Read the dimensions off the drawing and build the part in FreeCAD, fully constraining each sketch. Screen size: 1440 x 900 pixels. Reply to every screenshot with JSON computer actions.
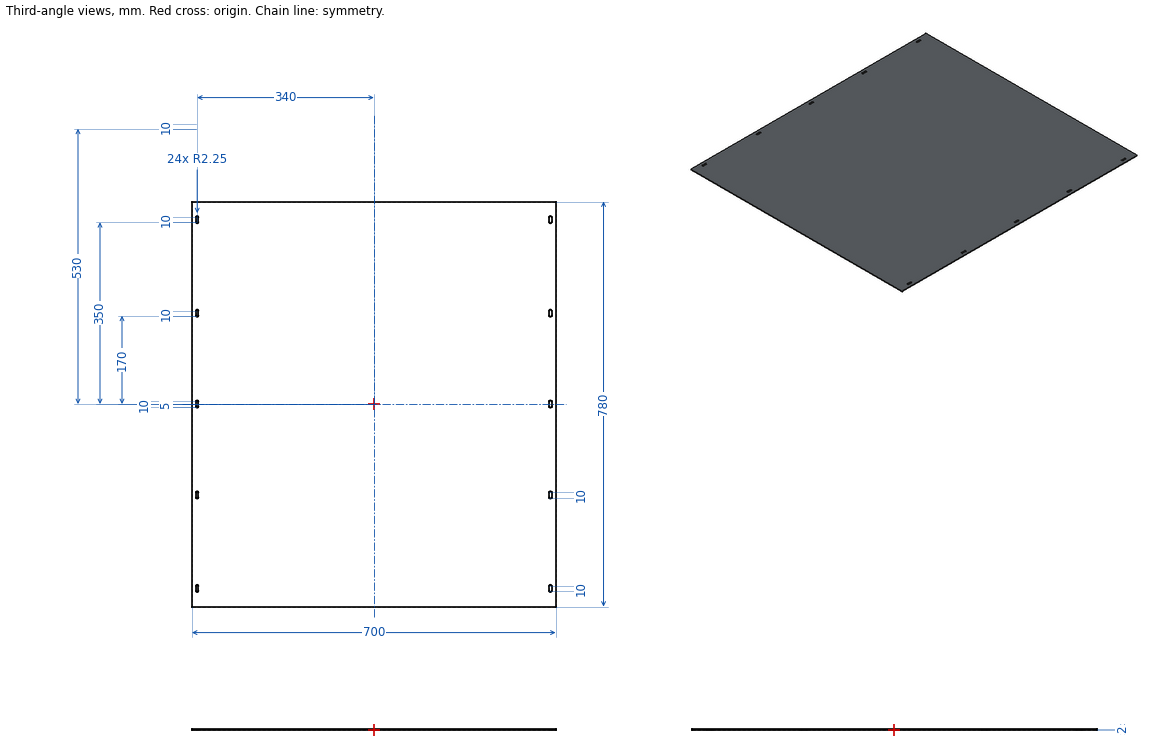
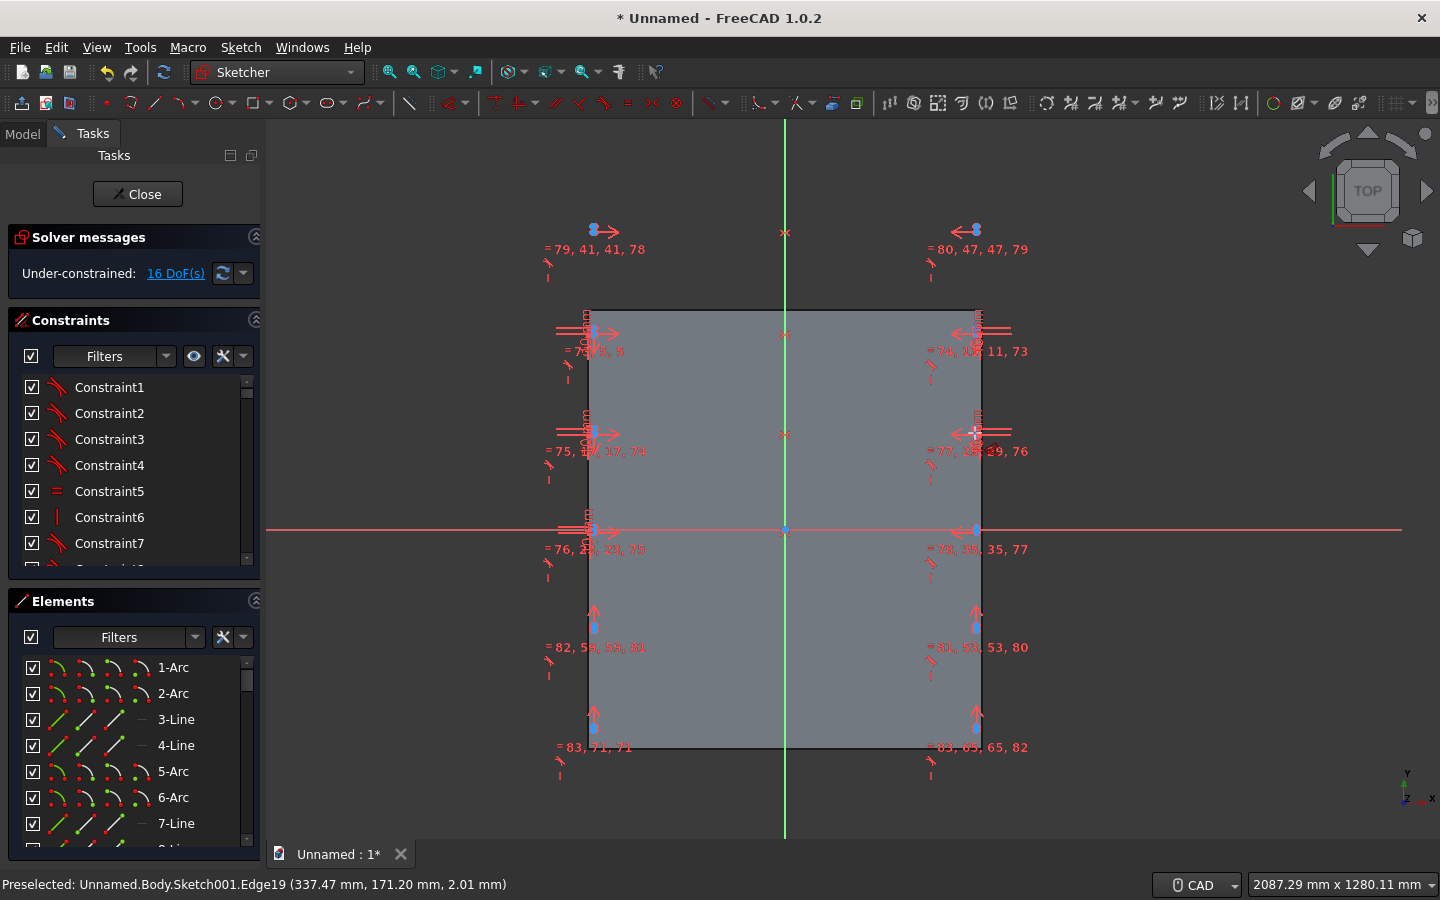
{"action": "scroll", "coordinate": [975, 531], "scroll_direction": "up", "scroll_amount": 12}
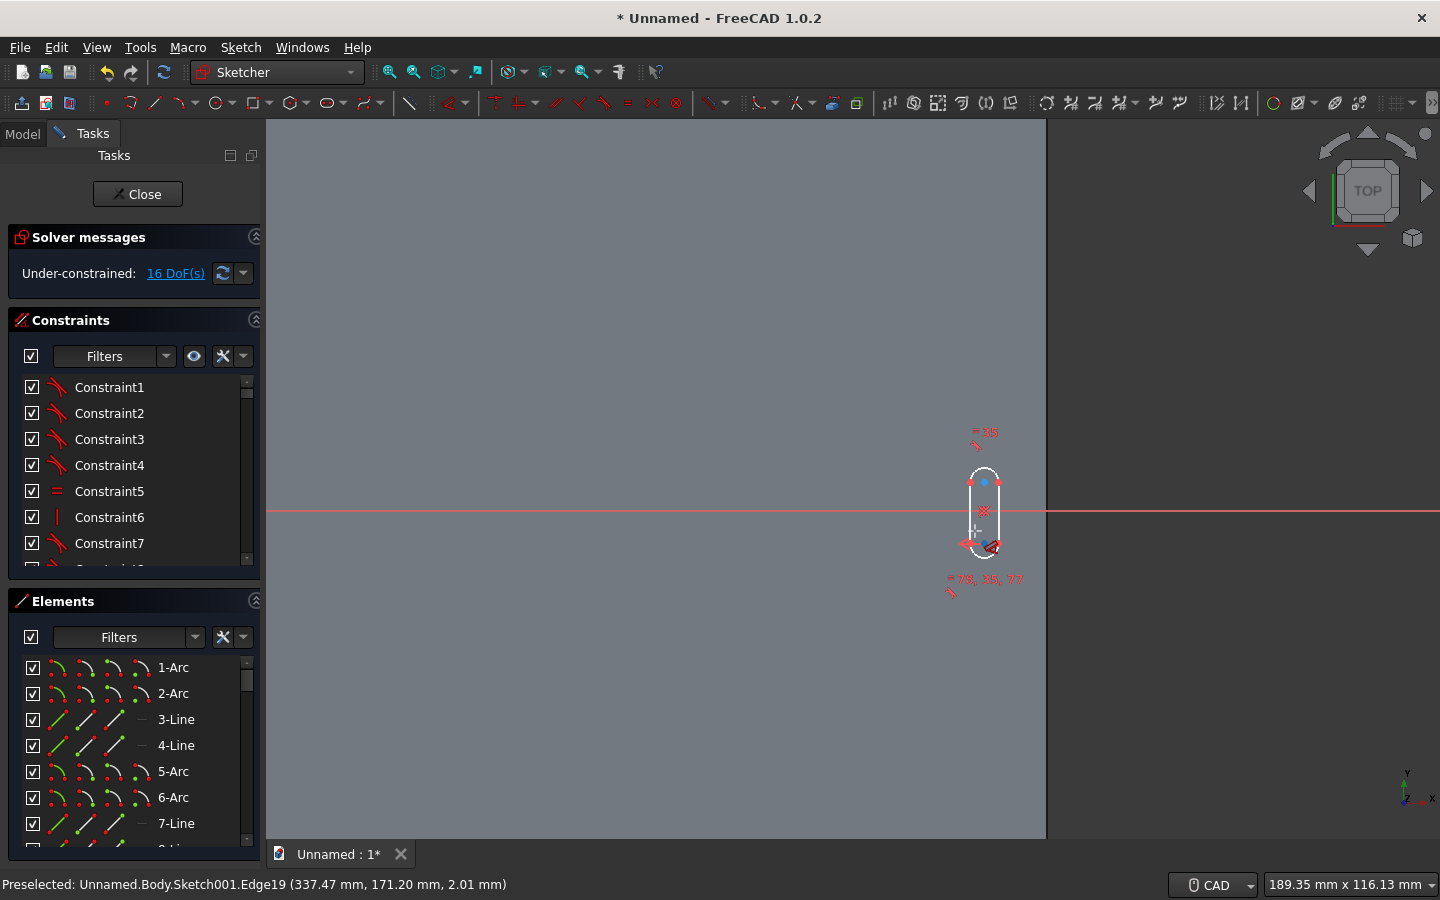
{"action": "left_click", "coordinate": [970, 525]}
{"action": "left_click", "coordinate": [936, 527]}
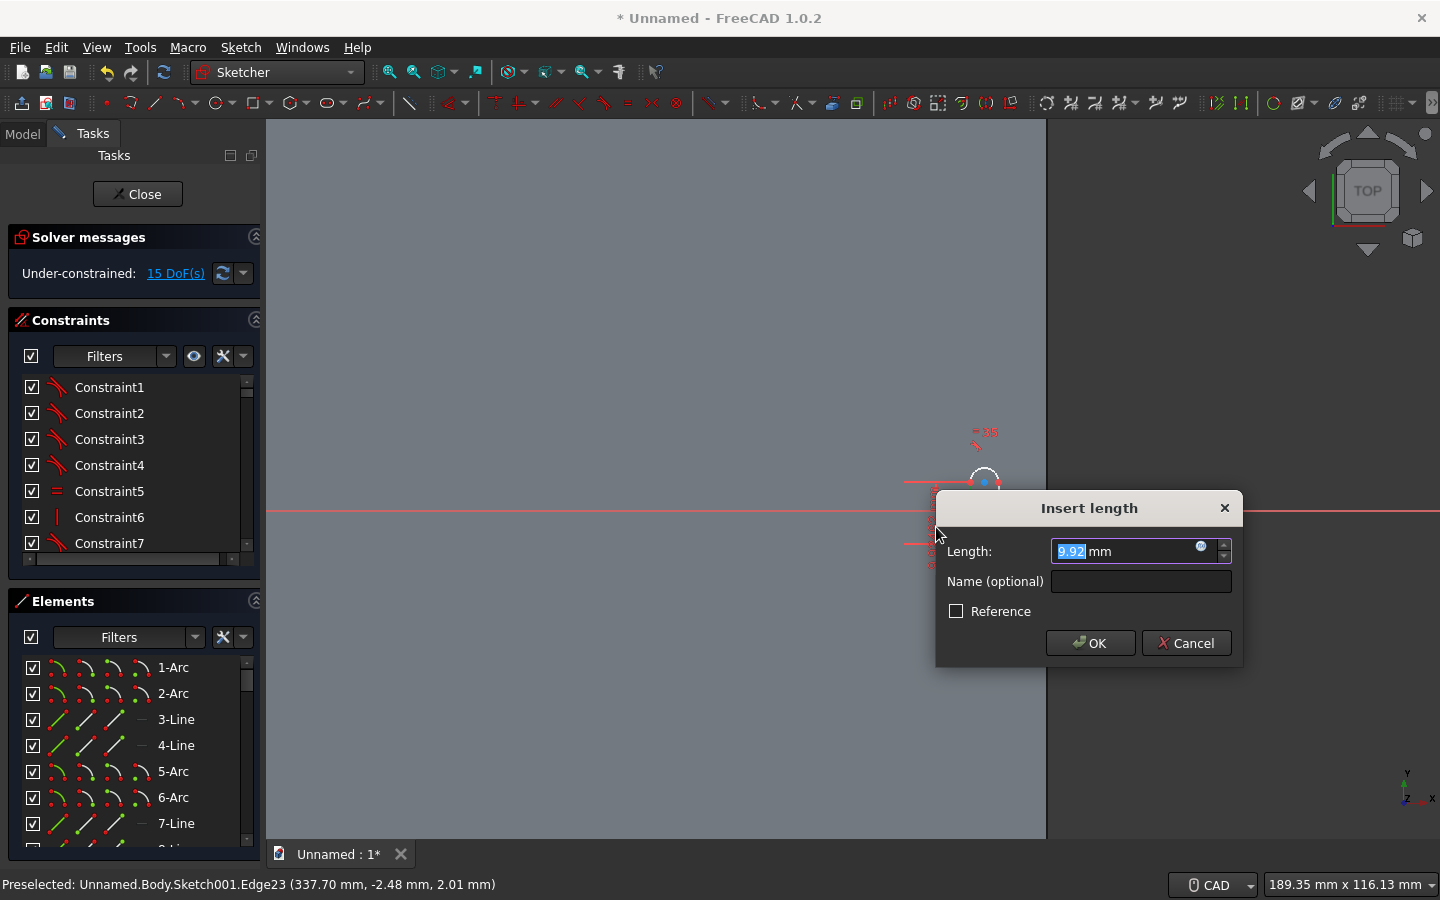
{"action": "type", "text": "10"}
{"action": "key", "text": "Return"}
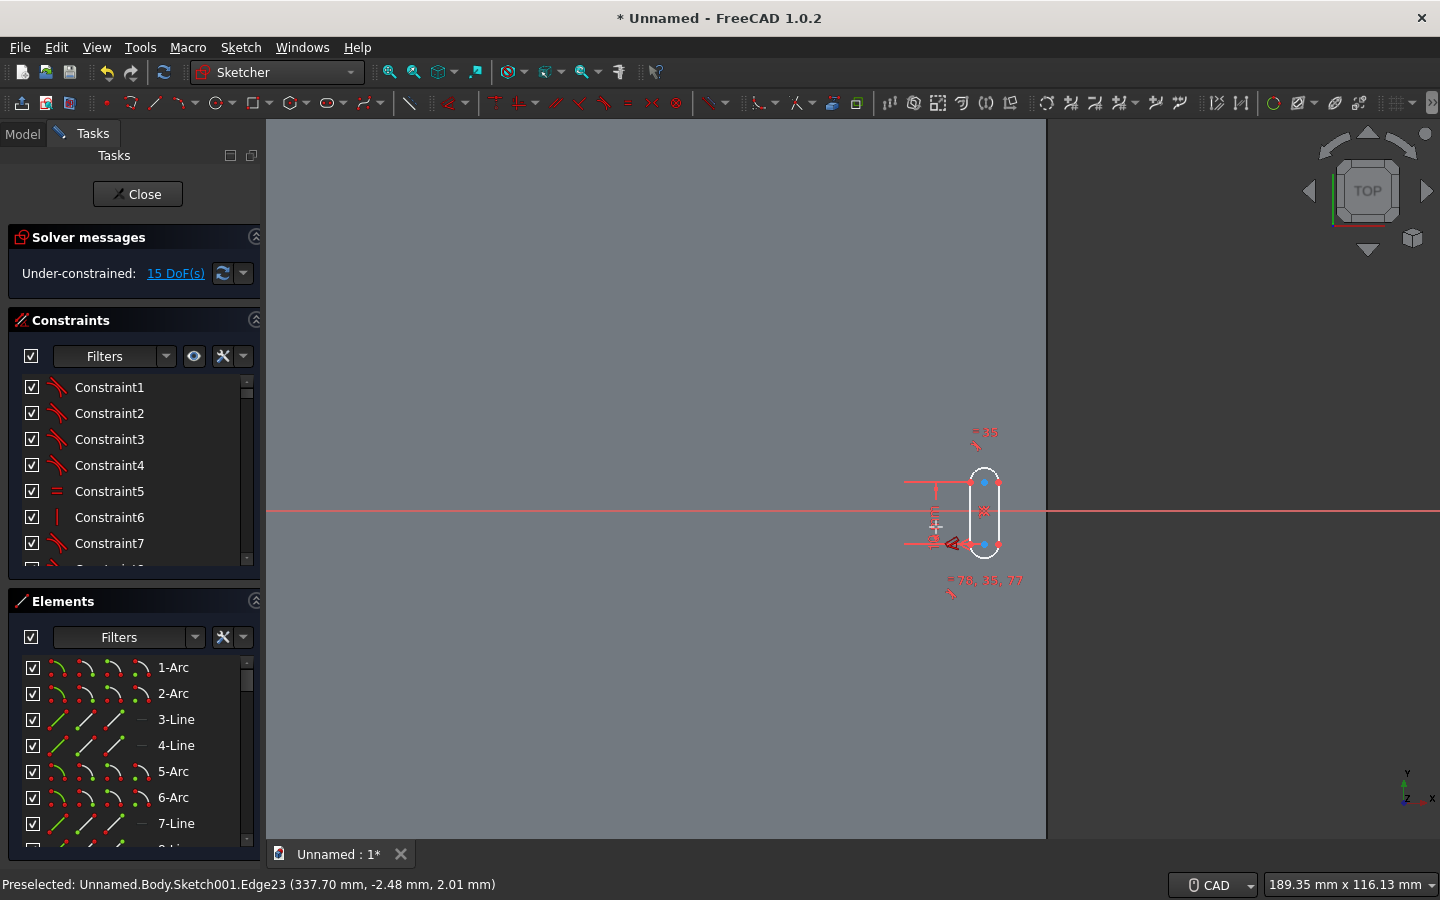
{"action": "scroll", "coordinate": [975, 532], "scroll_direction": "down", "scroll_amount": 12}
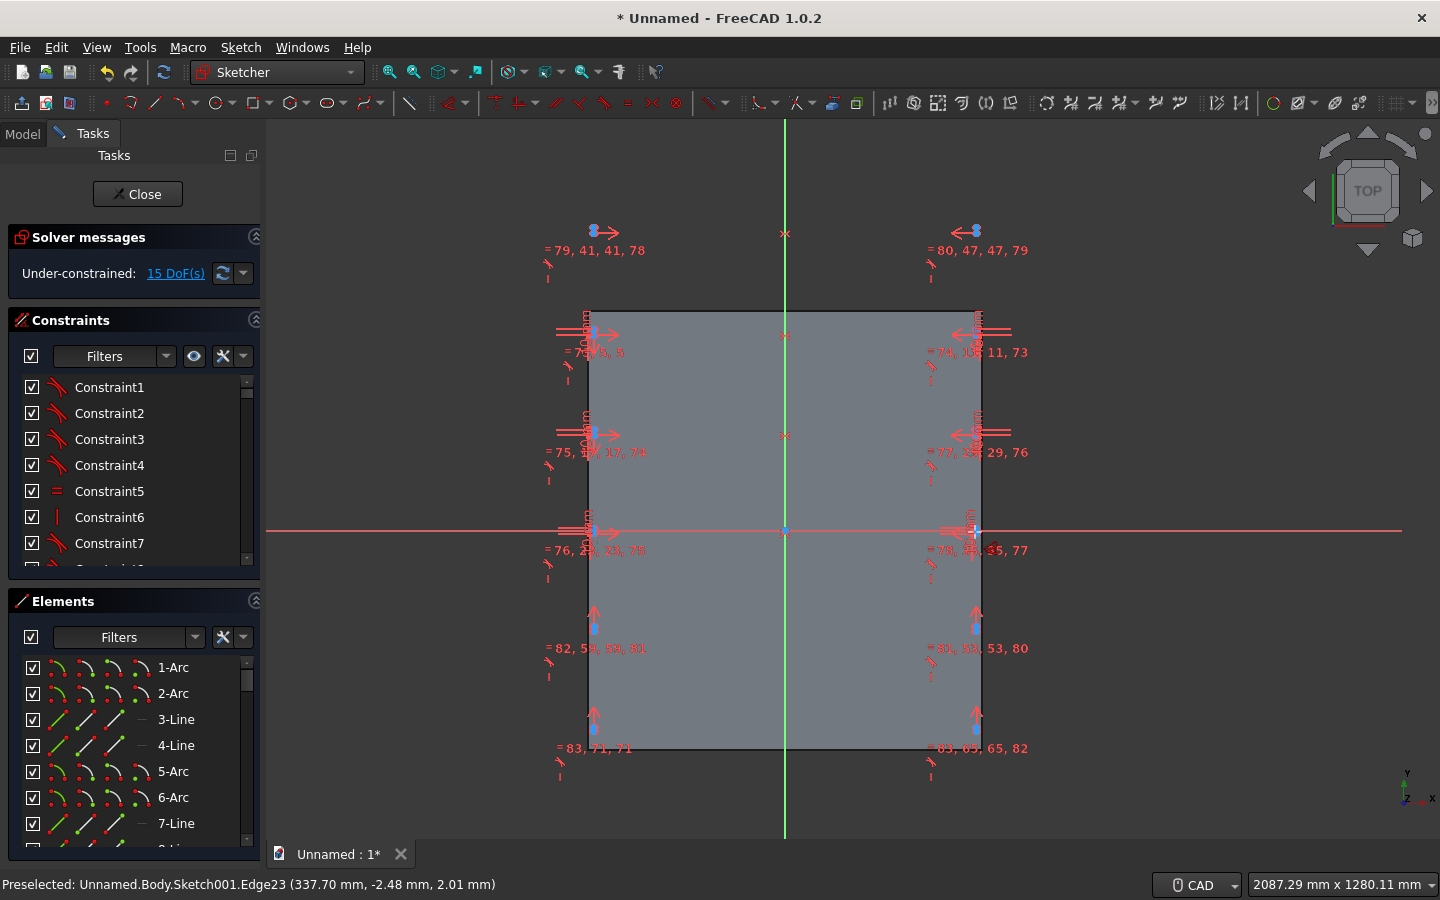
{"action": "scroll", "coordinate": [593, 231], "scroll_direction": "up", "scroll_amount": 11}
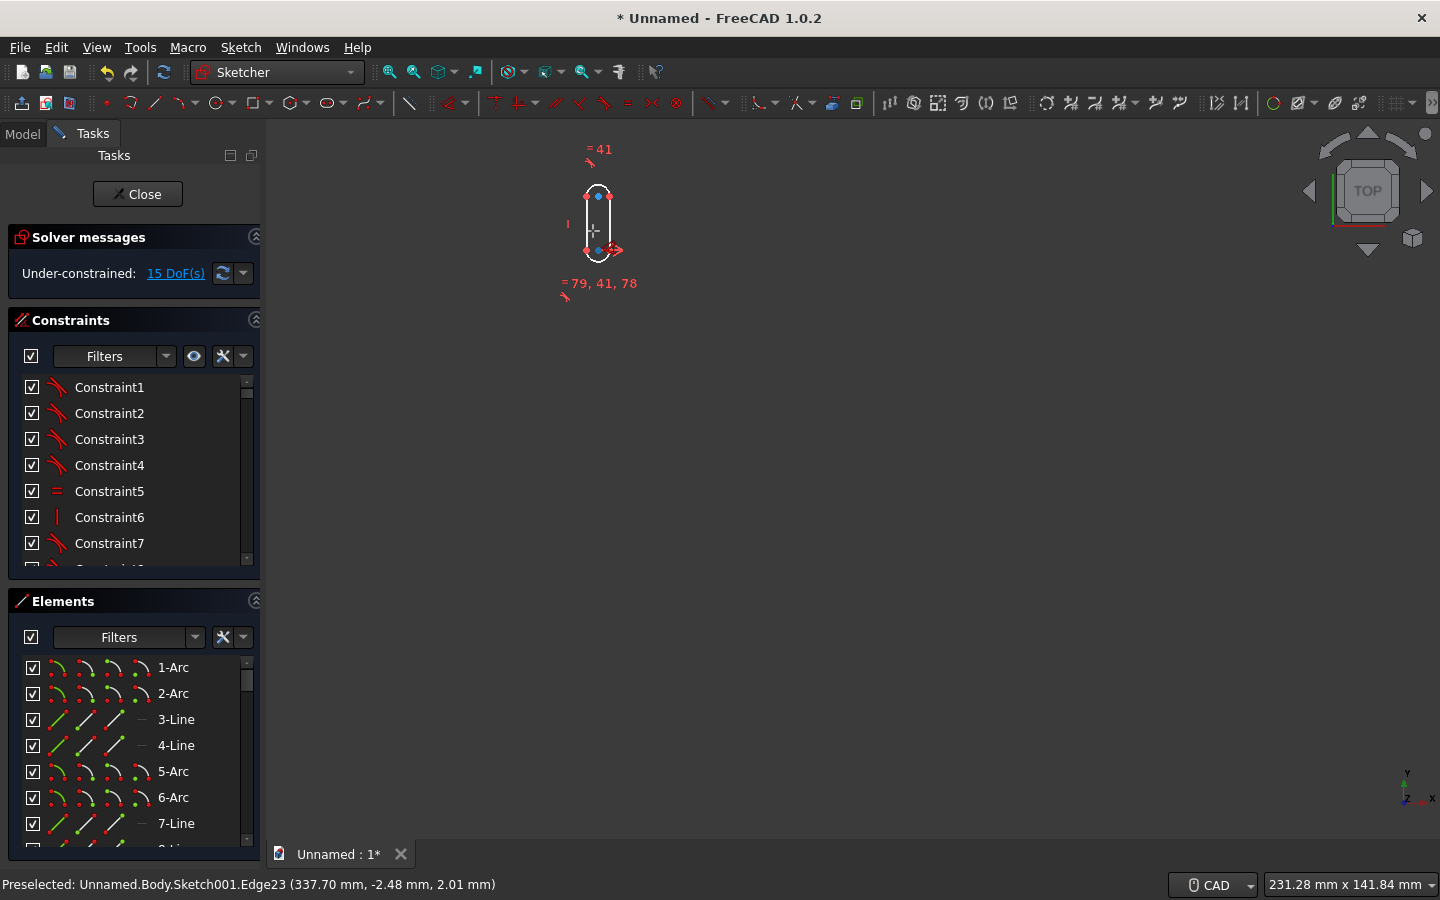
{"action": "left_click", "coordinate": [587, 234]}
{"action": "left_click", "coordinate": [553, 223]}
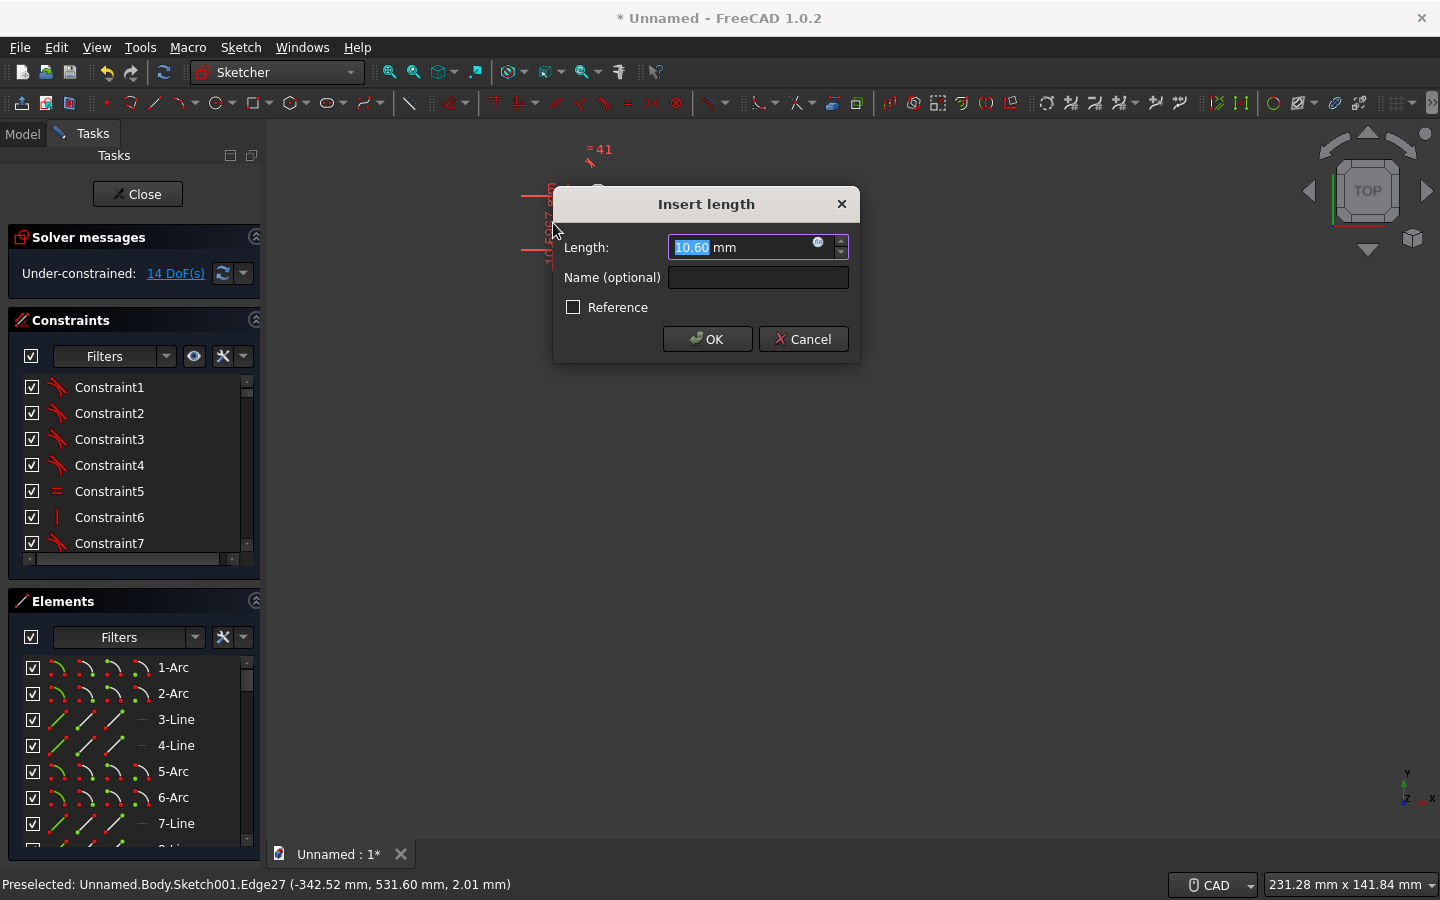
{"action": "type", "text": "10"}
{"action": "key", "text": "Return"}